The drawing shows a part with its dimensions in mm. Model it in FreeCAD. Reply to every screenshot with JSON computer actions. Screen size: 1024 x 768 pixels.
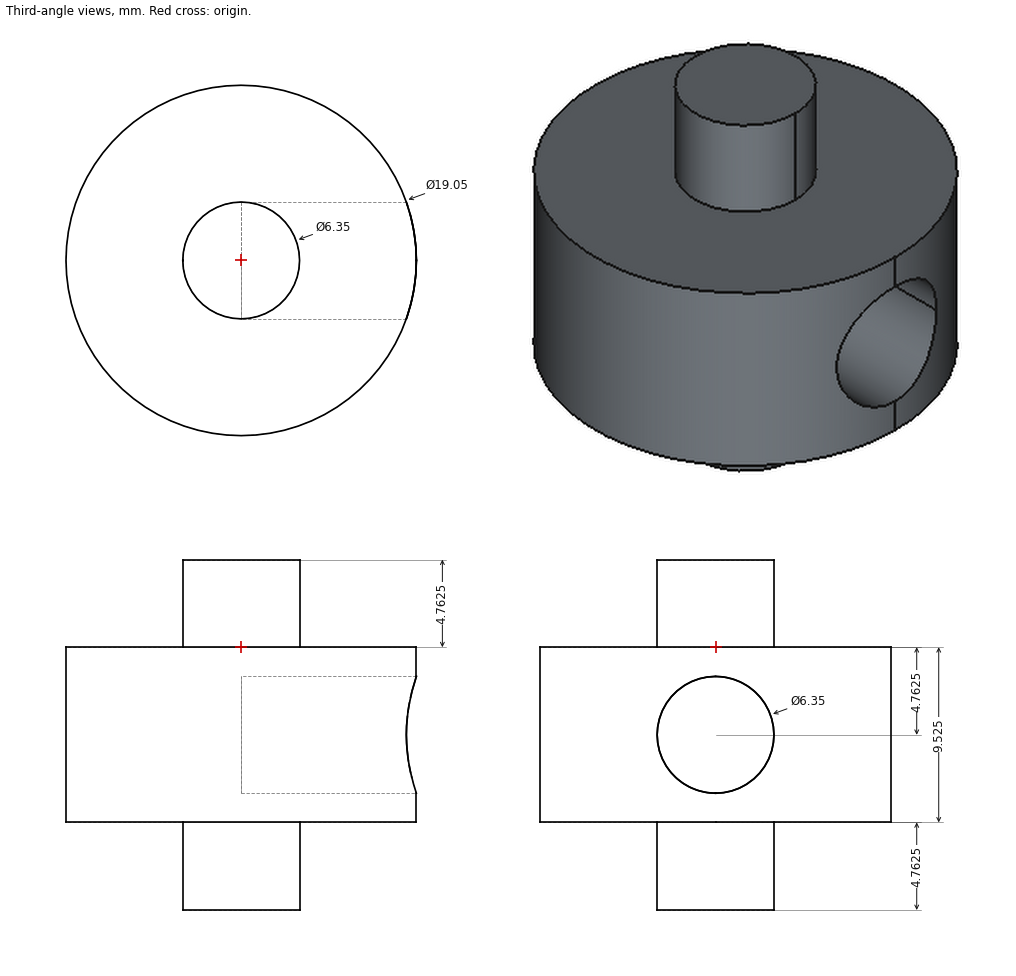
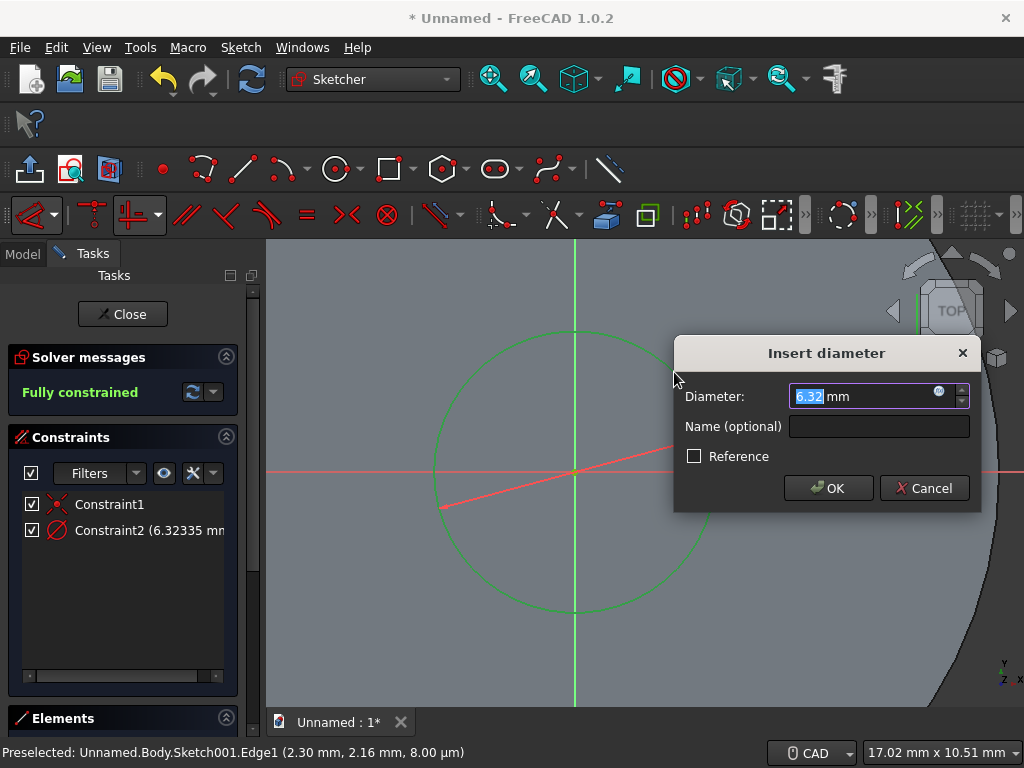
{"action": "type", "text": "6.35"}
{"action": "key", "text": "Return"}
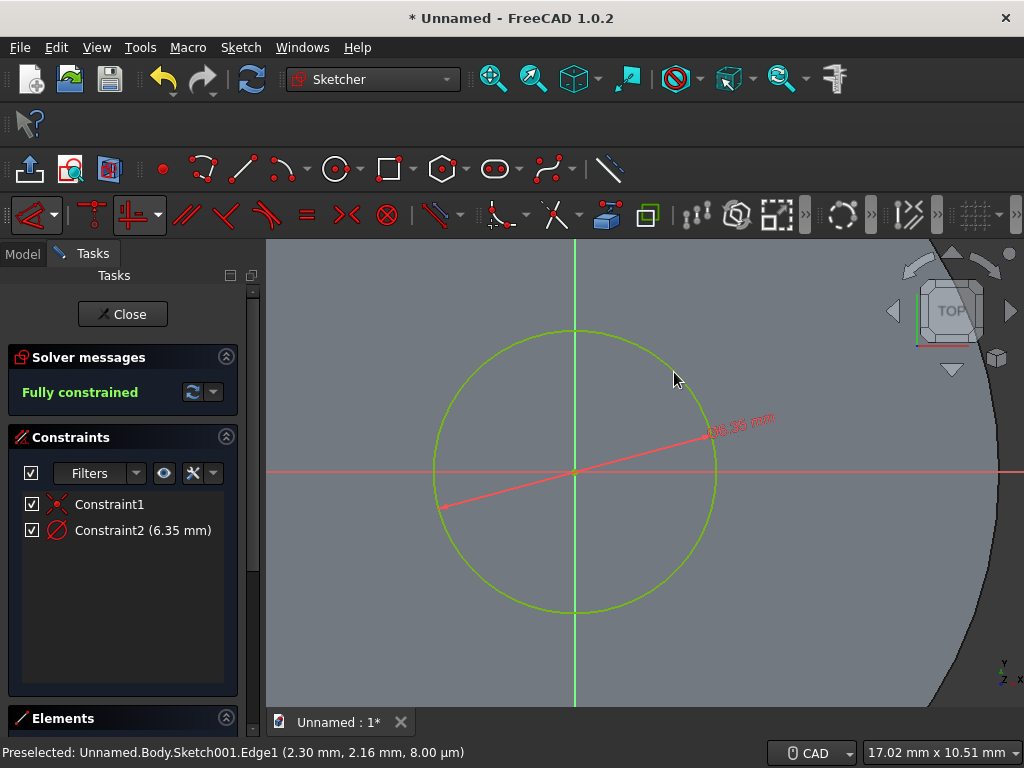
{"action": "left_click", "coordinate": [123, 314]}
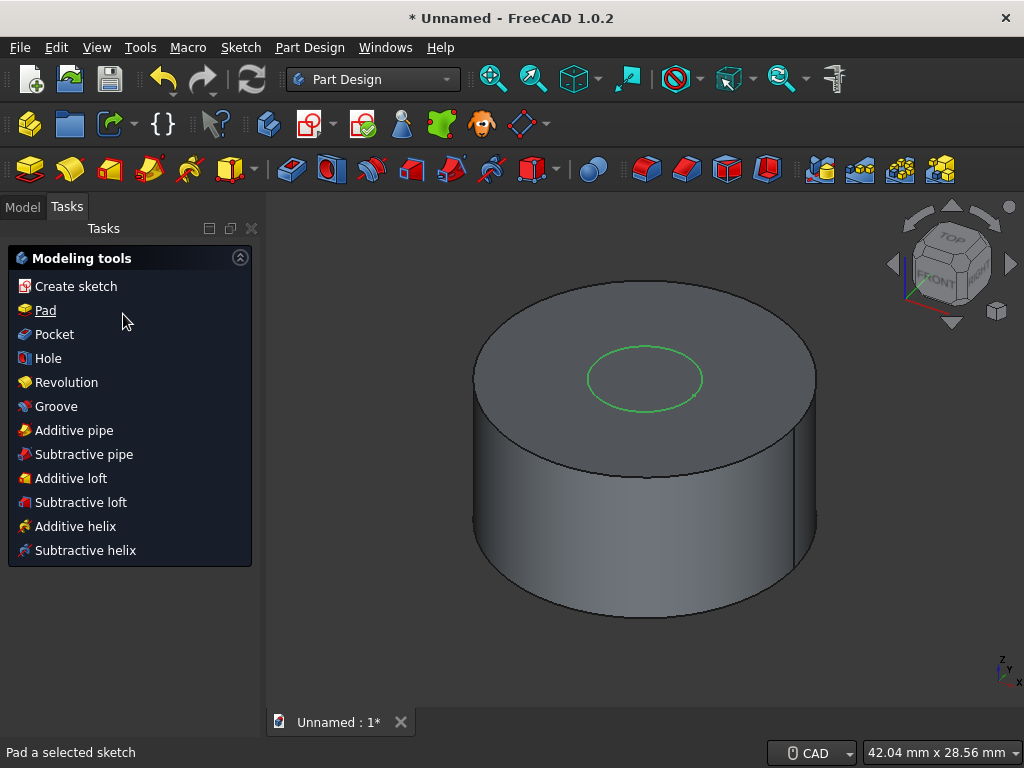
{"action": "left_click", "coordinate": [30, 170]}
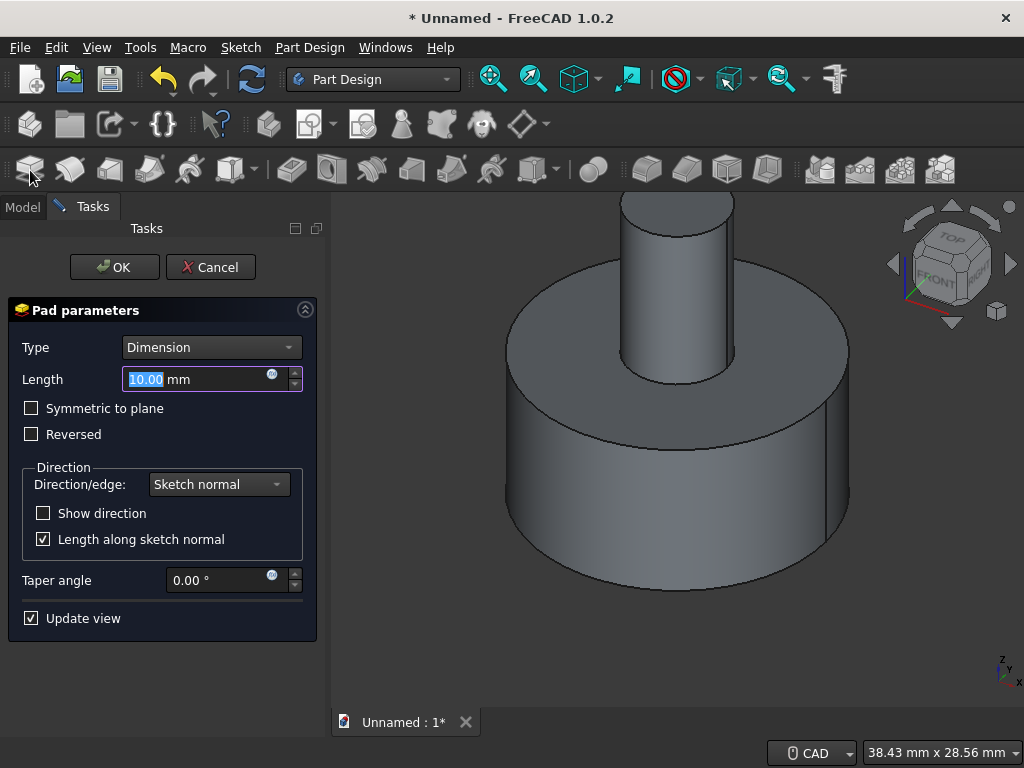
{"action": "type", "text": "4.7625"}
{"action": "key", "text": "Tab"}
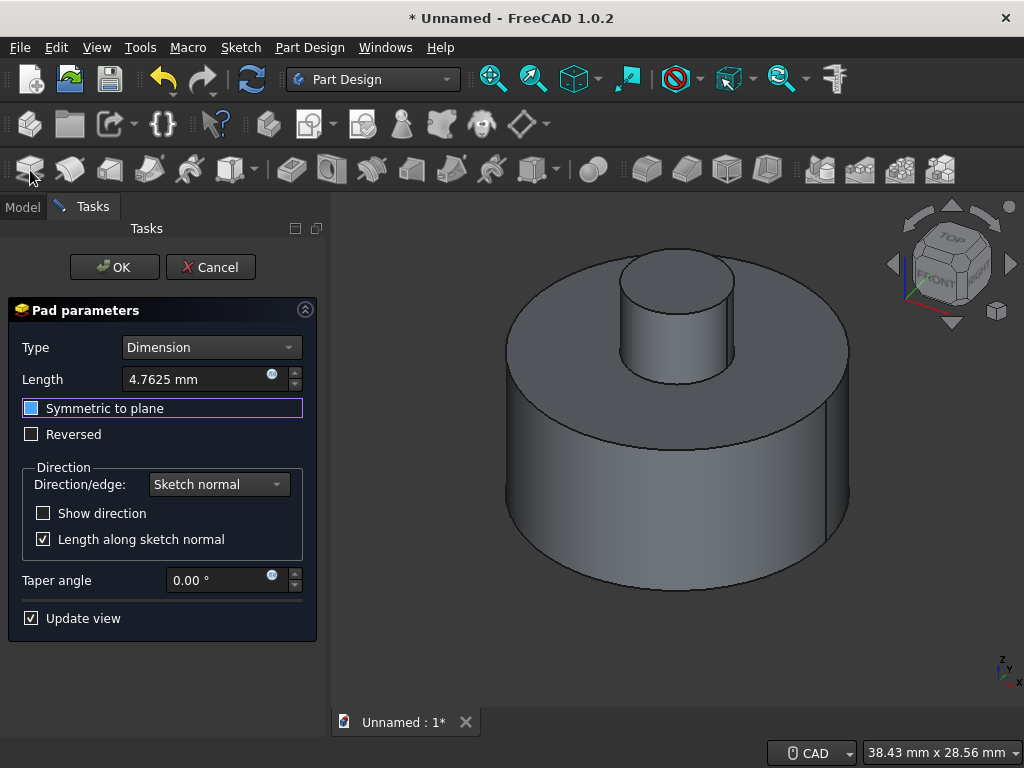
{"action": "left_click", "coordinate": [115, 267]}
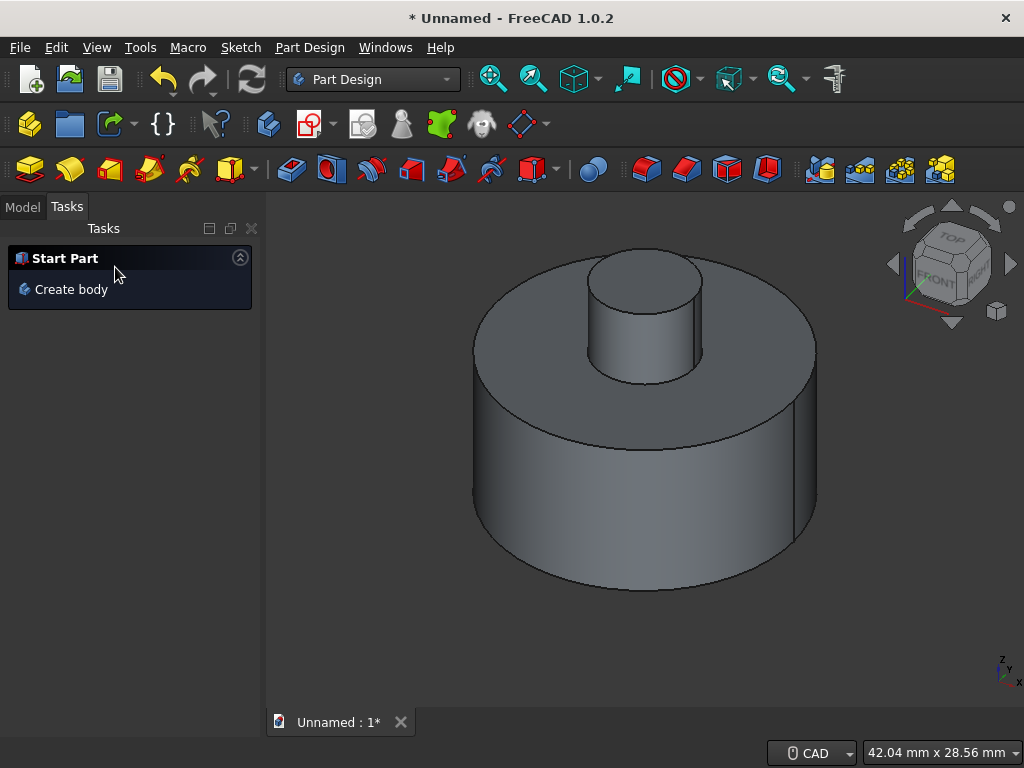
{"action": "key", "text": "v f"}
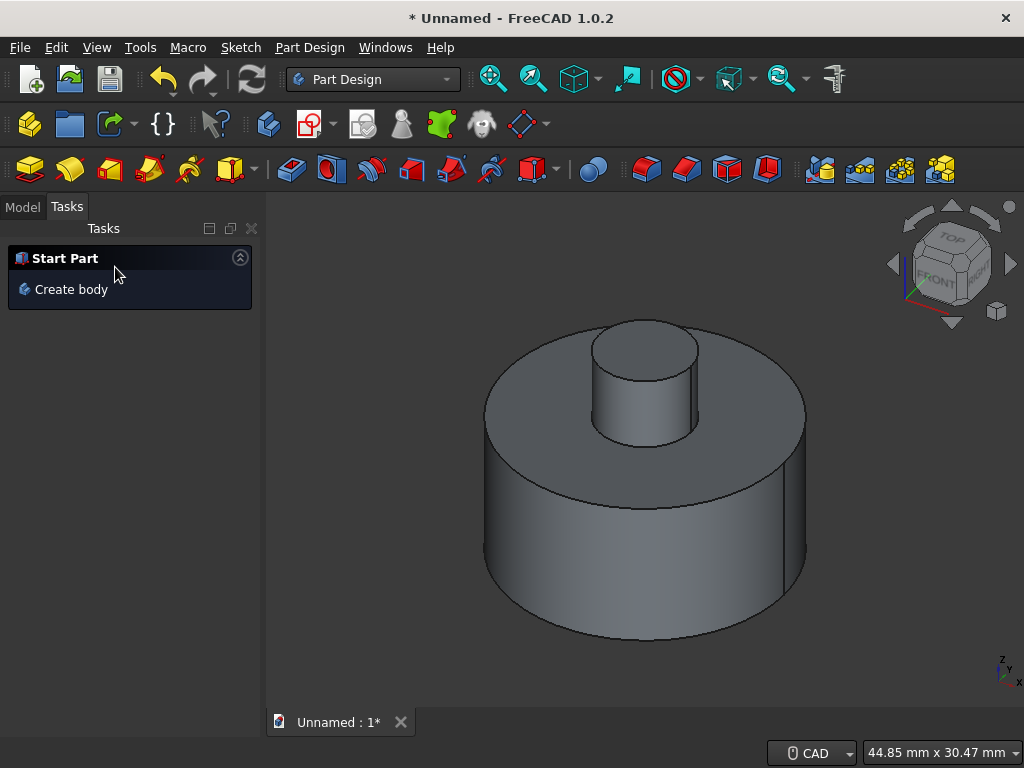
{"action": "left_click", "coordinate": [23, 206]}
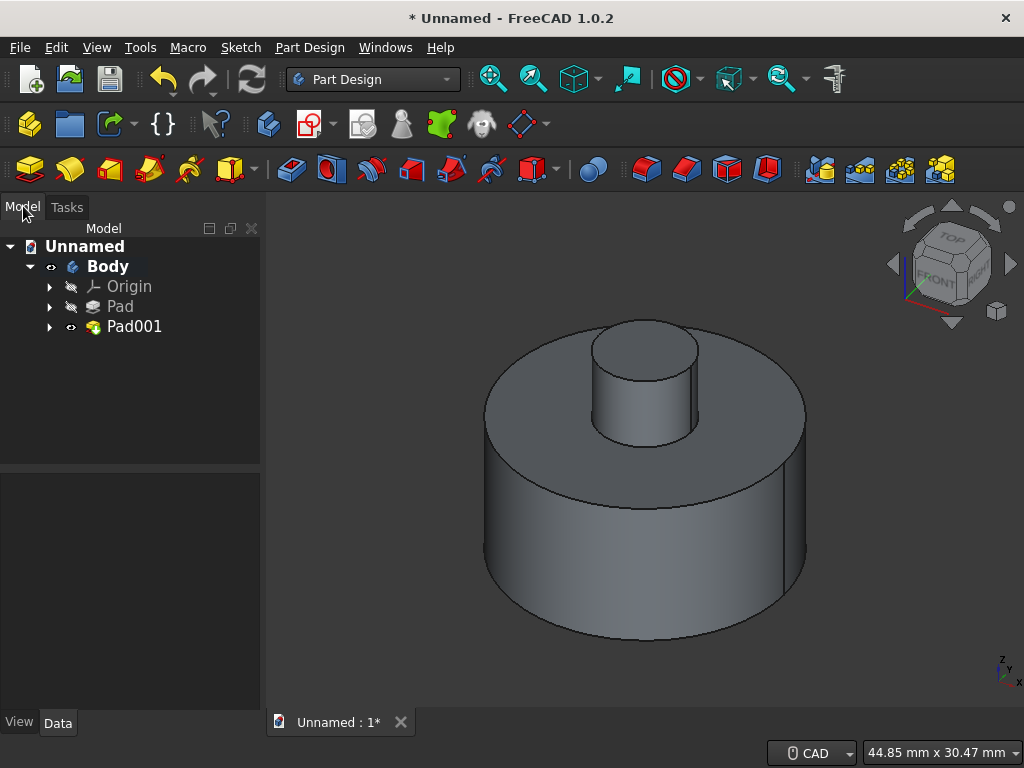
{"action": "left_click", "coordinate": [50, 287]}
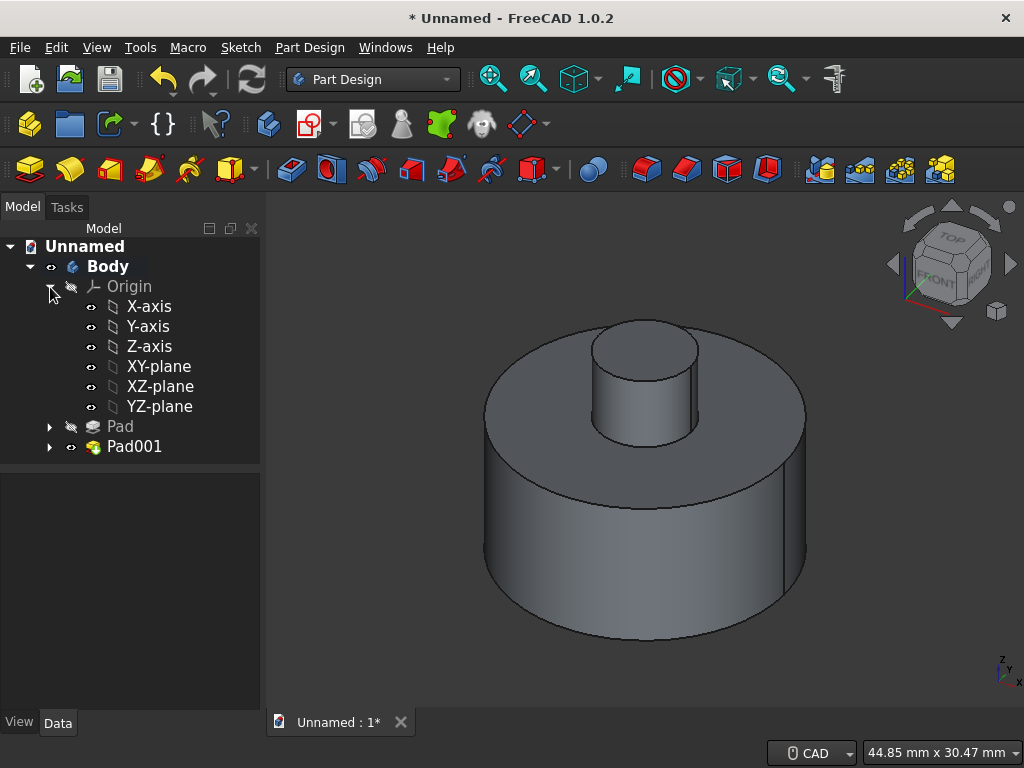
{"action": "left_click", "coordinate": [136, 367]}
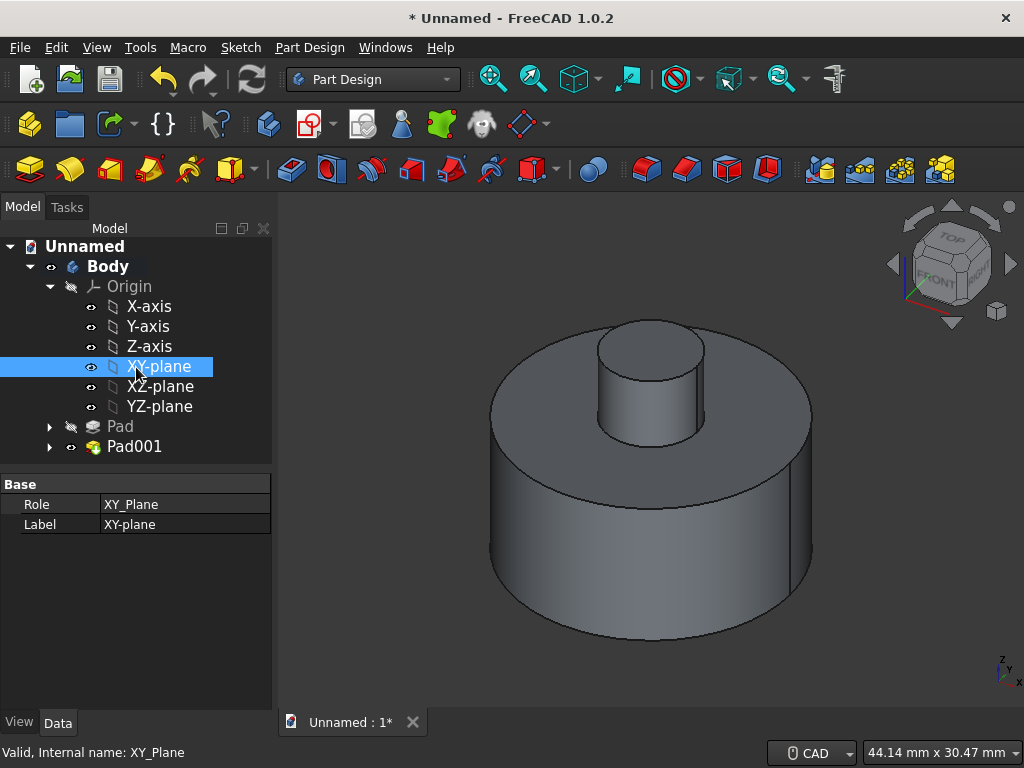
{"action": "left_click", "coordinate": [522, 124]}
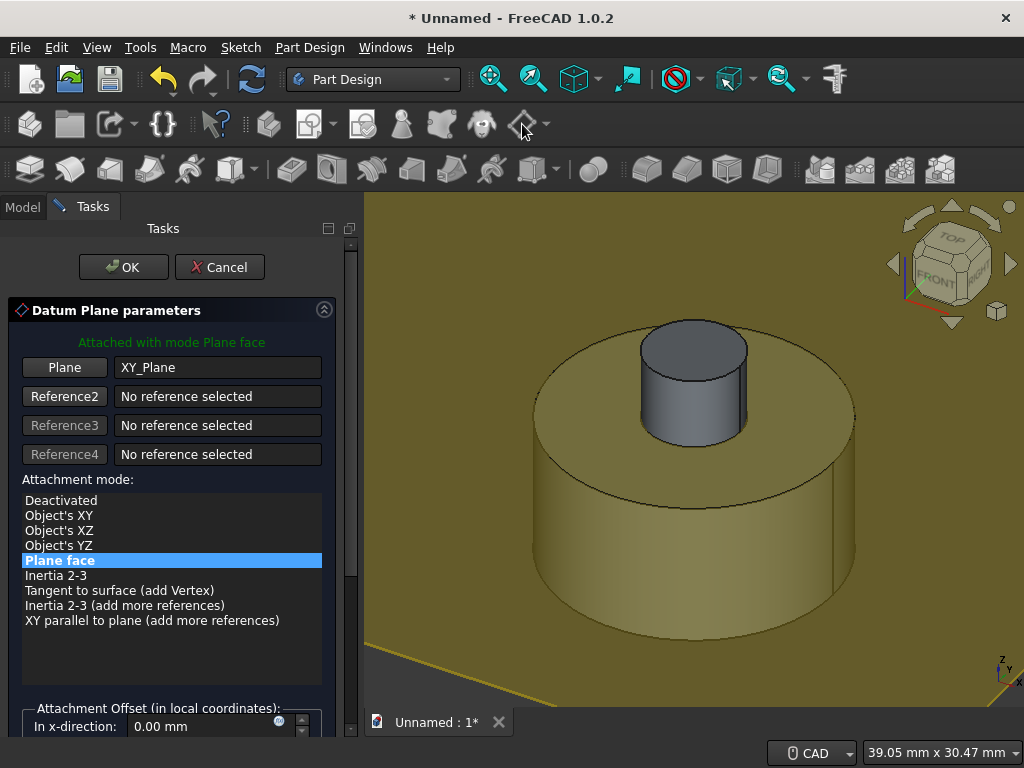
{"action": "scroll", "coordinate": [351, 487], "scroll_direction": "down", "scroll_amount": 3}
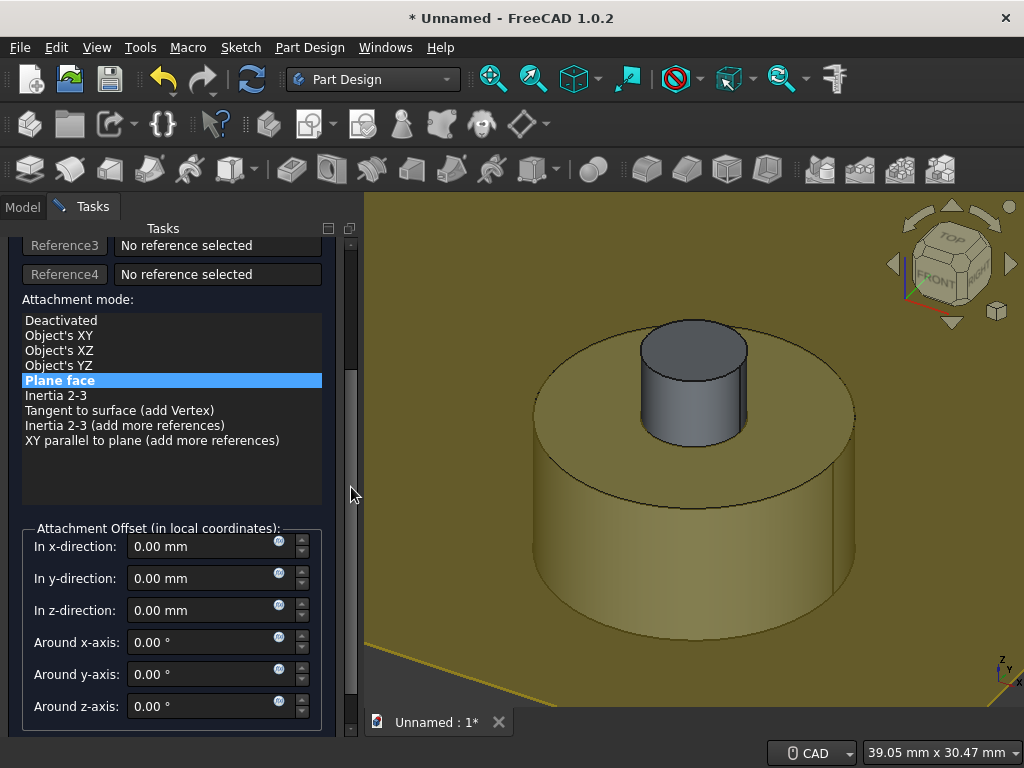
{"action": "triple_click", "coordinate": [210, 610]}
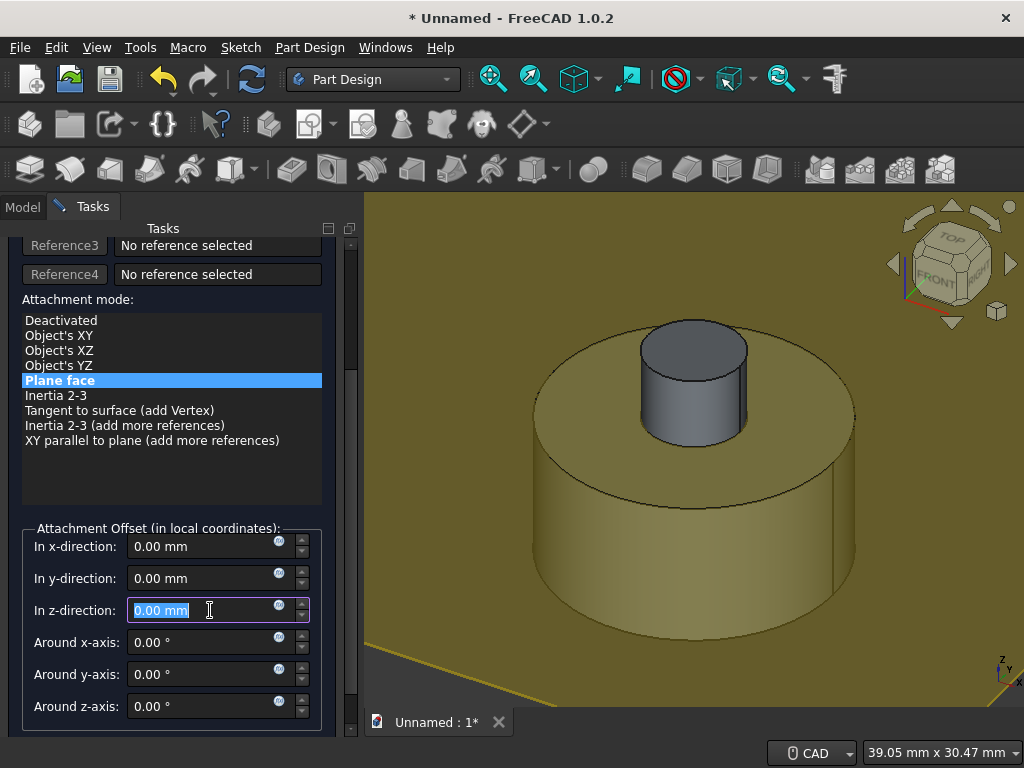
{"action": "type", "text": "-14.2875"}
{"action": "key", "text": "Tab"}